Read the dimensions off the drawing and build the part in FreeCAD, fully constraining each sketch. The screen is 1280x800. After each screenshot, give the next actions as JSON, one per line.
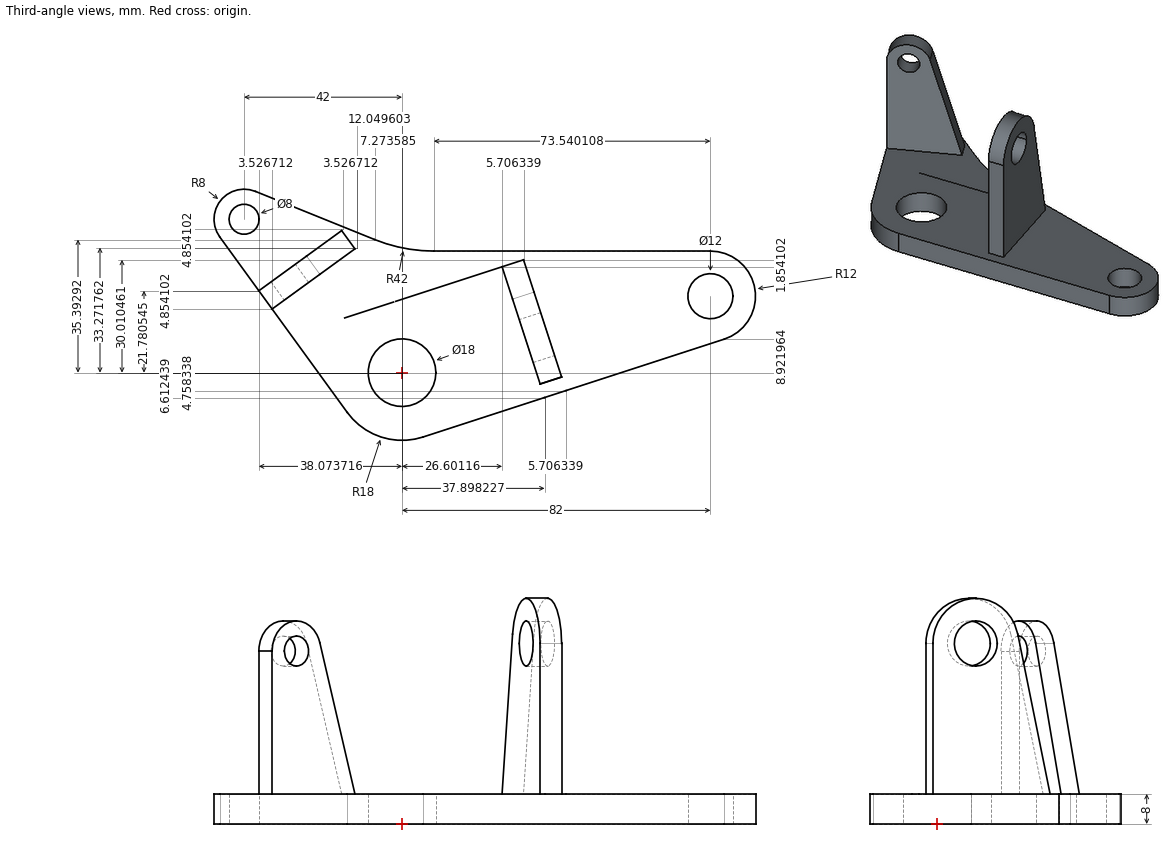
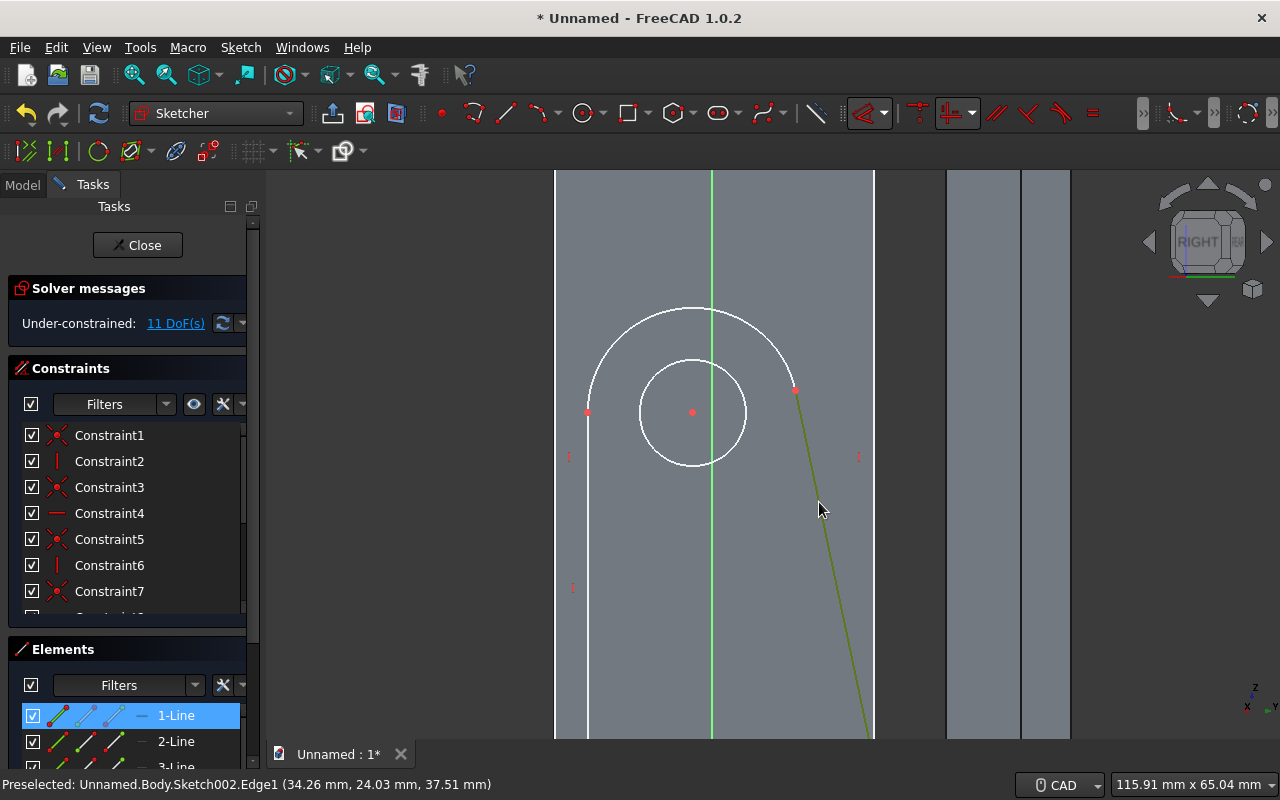
{"action": "left_click", "coordinate": [741, 320]}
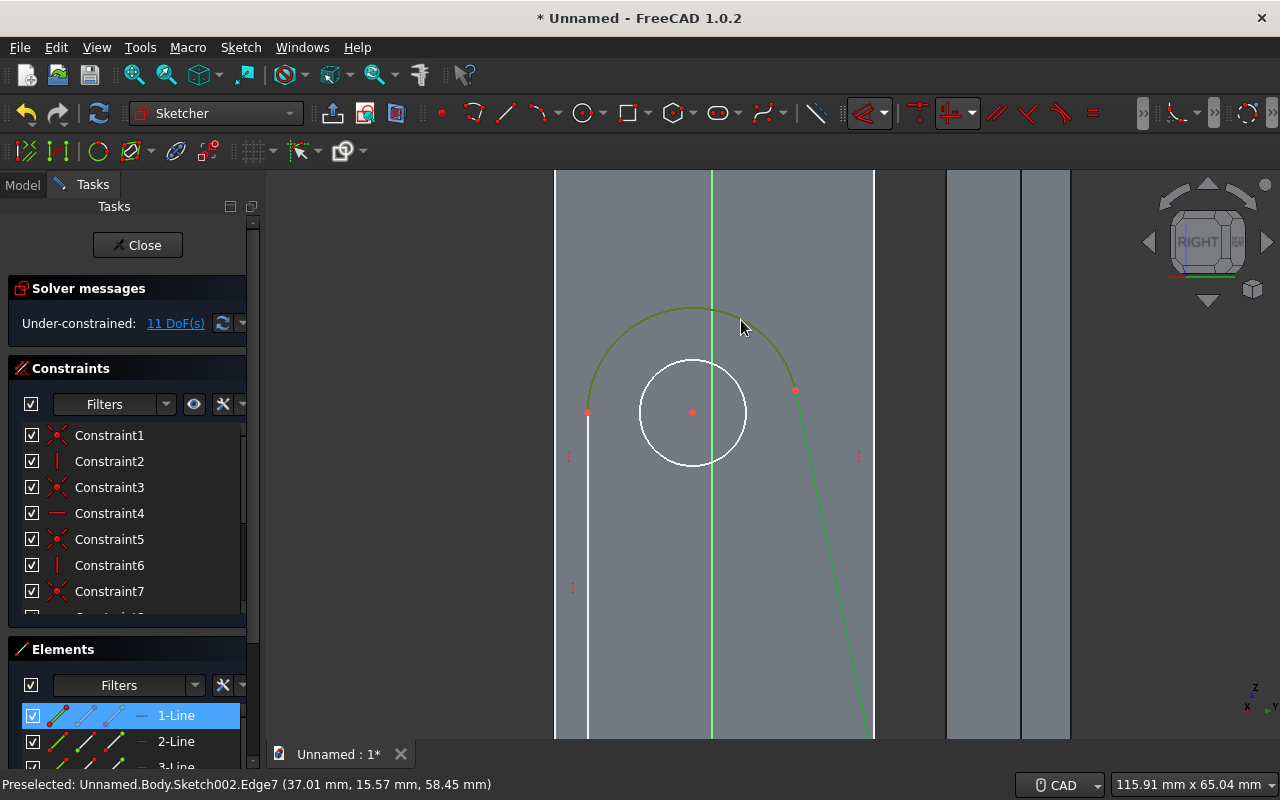
{"action": "key", "text": "t"}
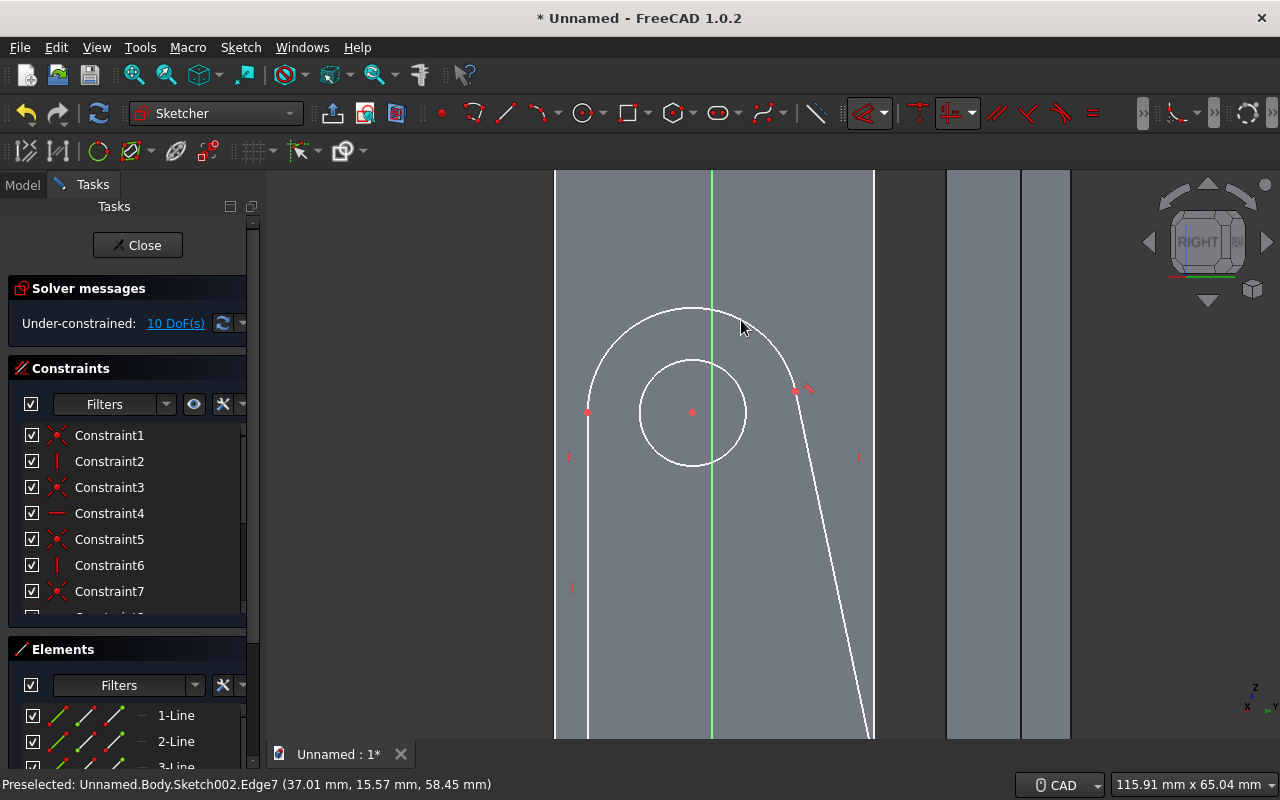
{"action": "left_click", "coordinate": [588, 657]}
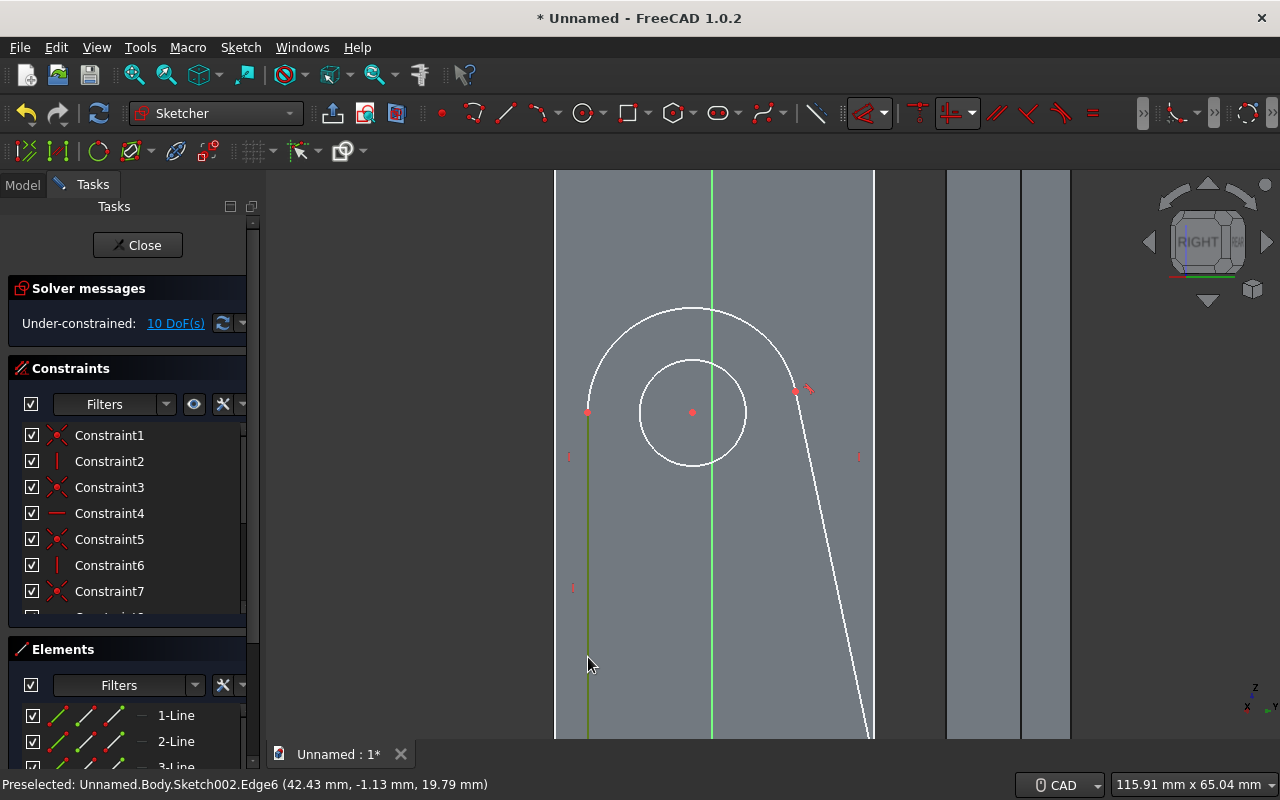
{"action": "left_click", "coordinate": [742, 320]}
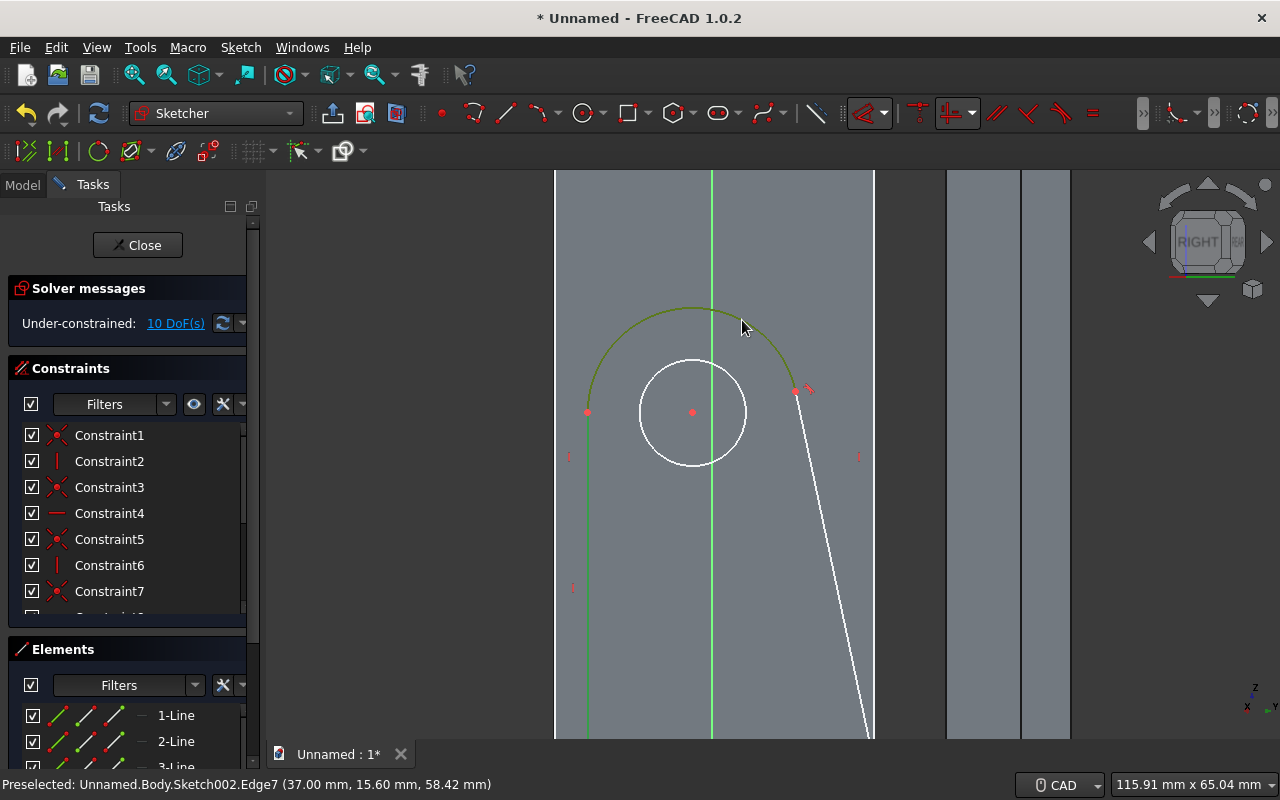
{"action": "left_click", "coordinate": [1062, 114]}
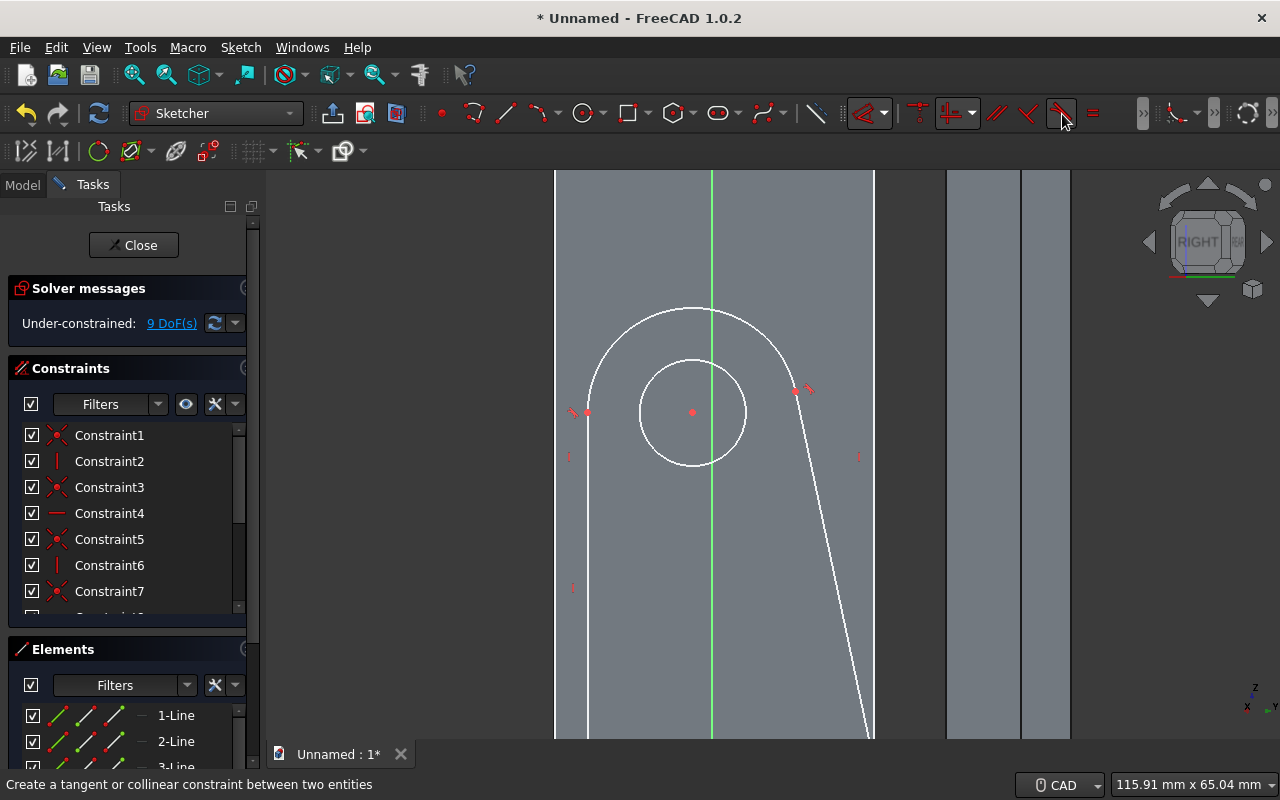
{"action": "left_click", "coordinate": [742, 320]}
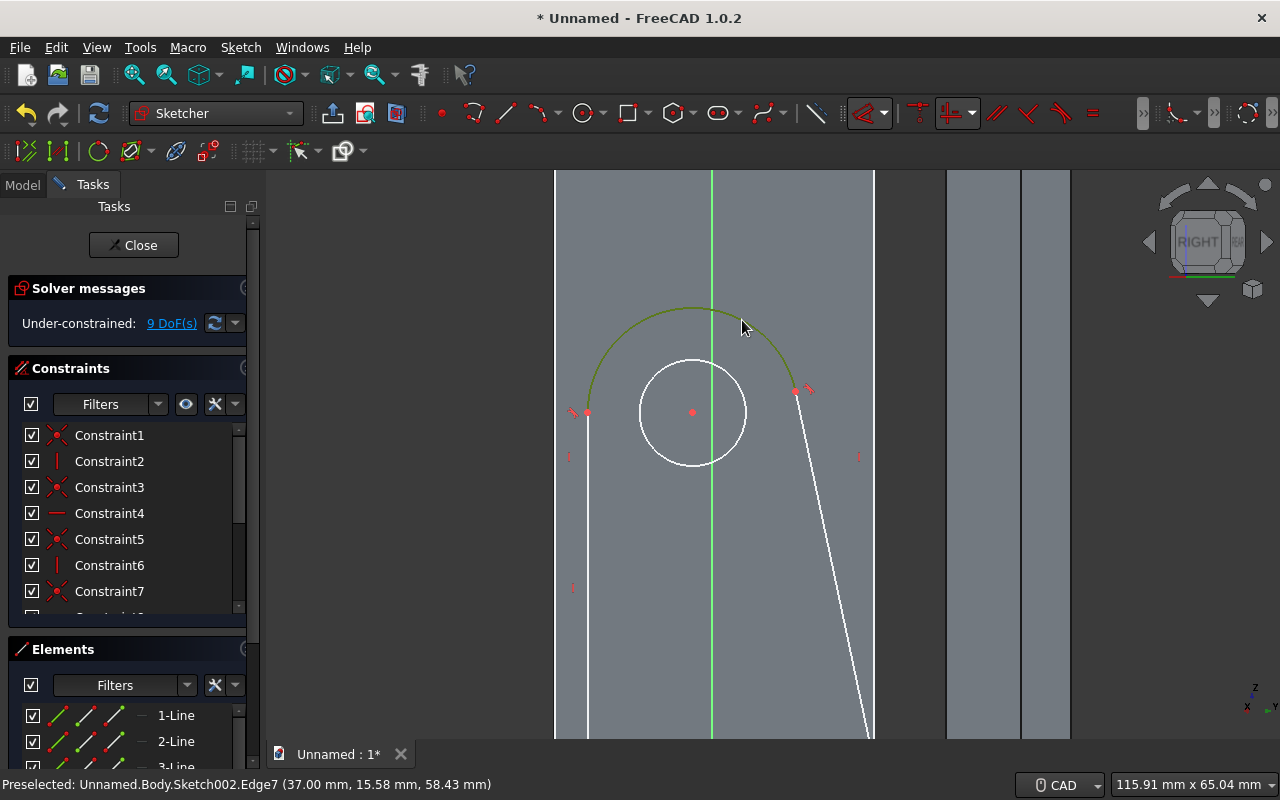
{"action": "left_click", "coordinate": [886, 114]}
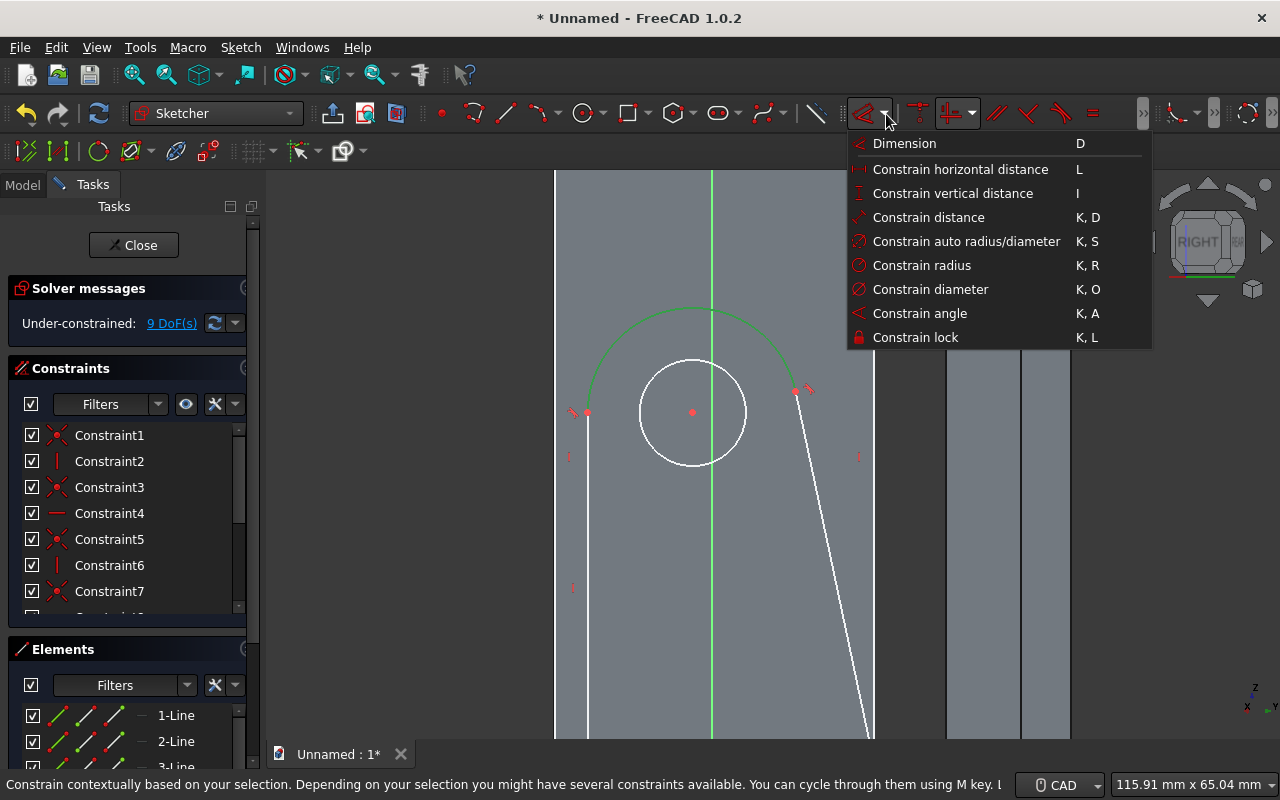
{"action": "left_click", "coordinate": [1000, 265]}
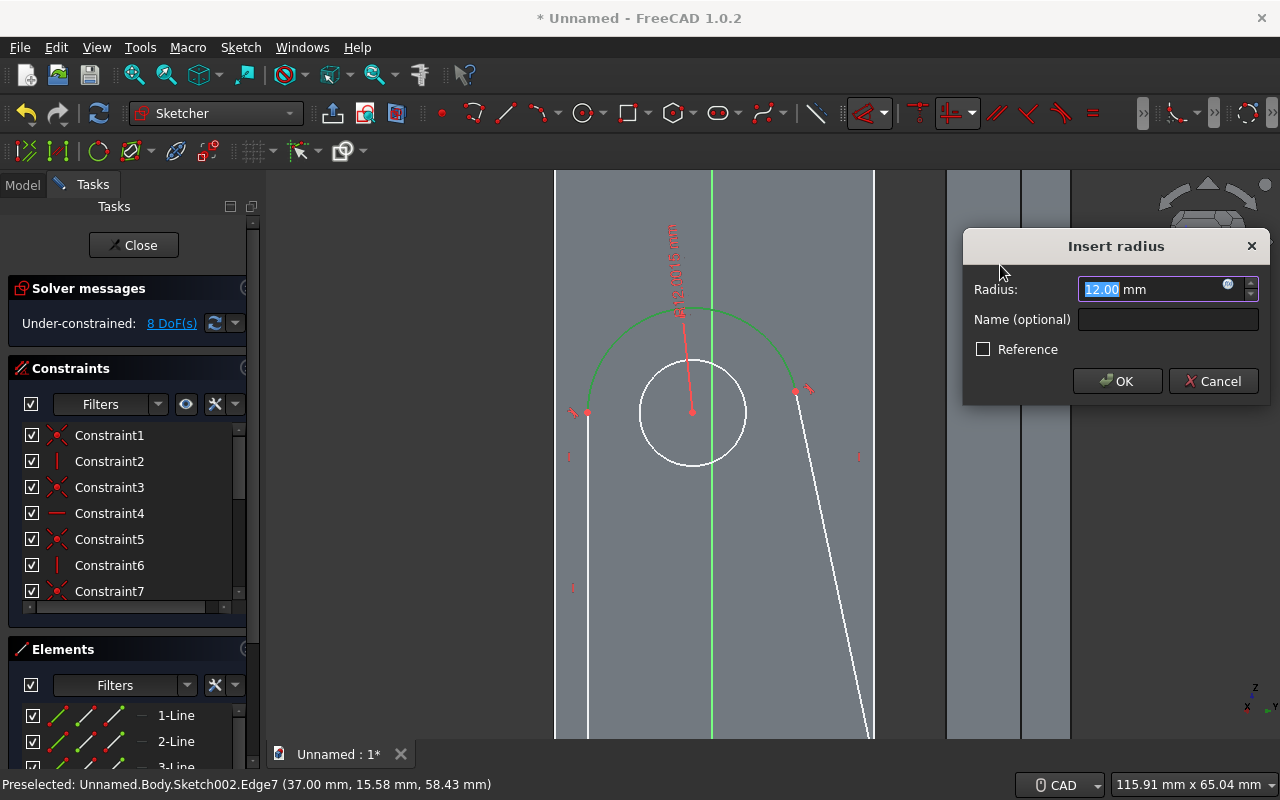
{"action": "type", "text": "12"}
{"action": "key", "text": "Return"}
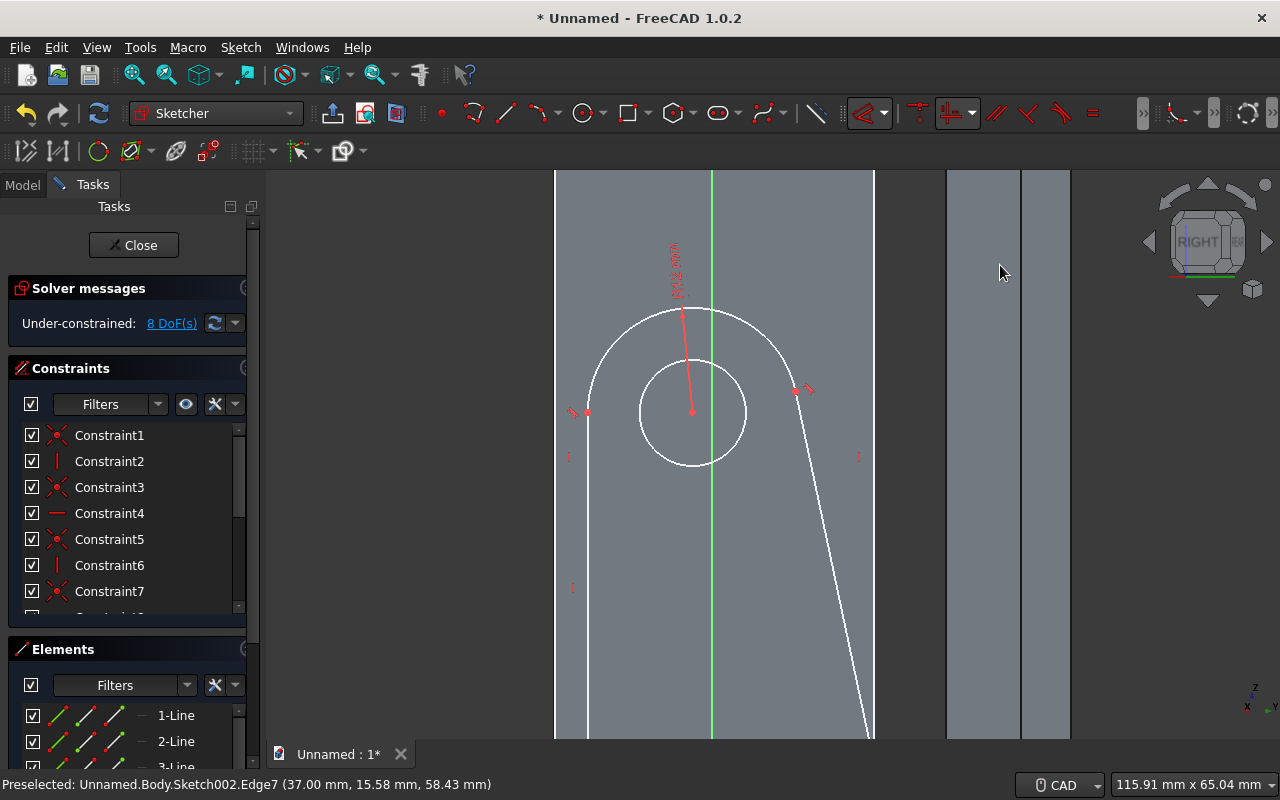
{"action": "left_click", "coordinate": [730, 375]}